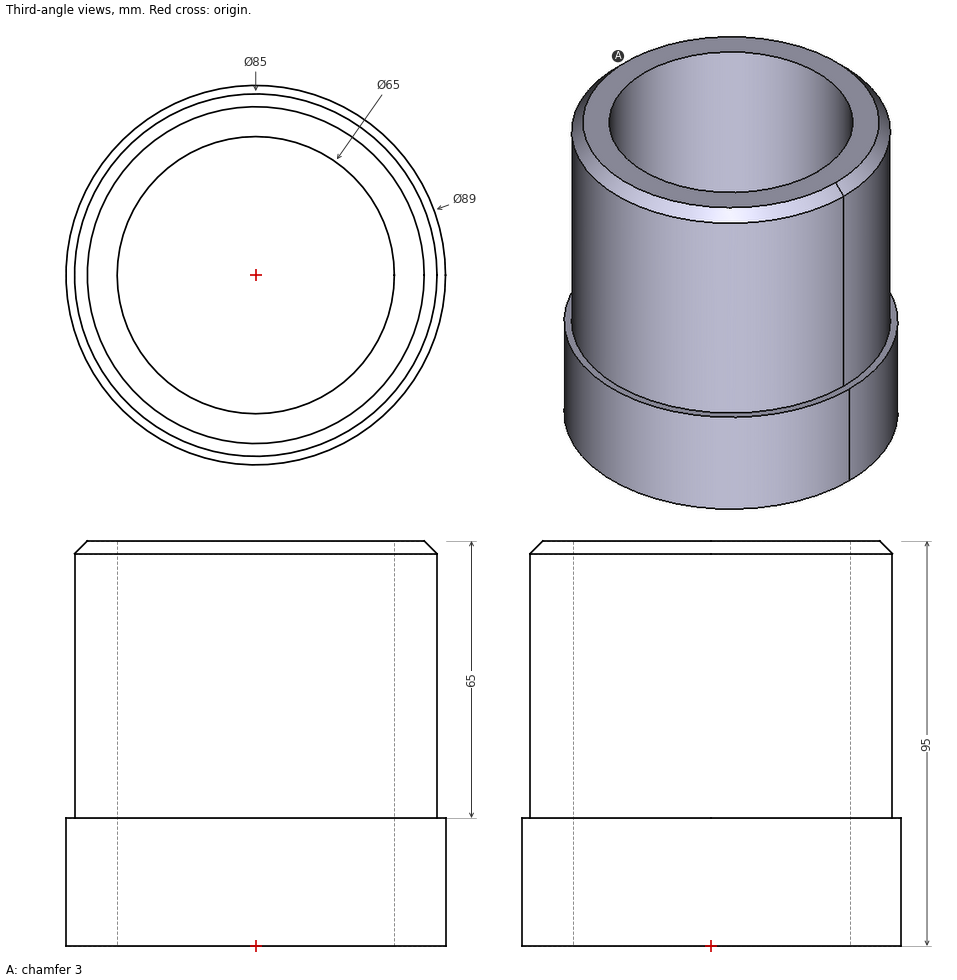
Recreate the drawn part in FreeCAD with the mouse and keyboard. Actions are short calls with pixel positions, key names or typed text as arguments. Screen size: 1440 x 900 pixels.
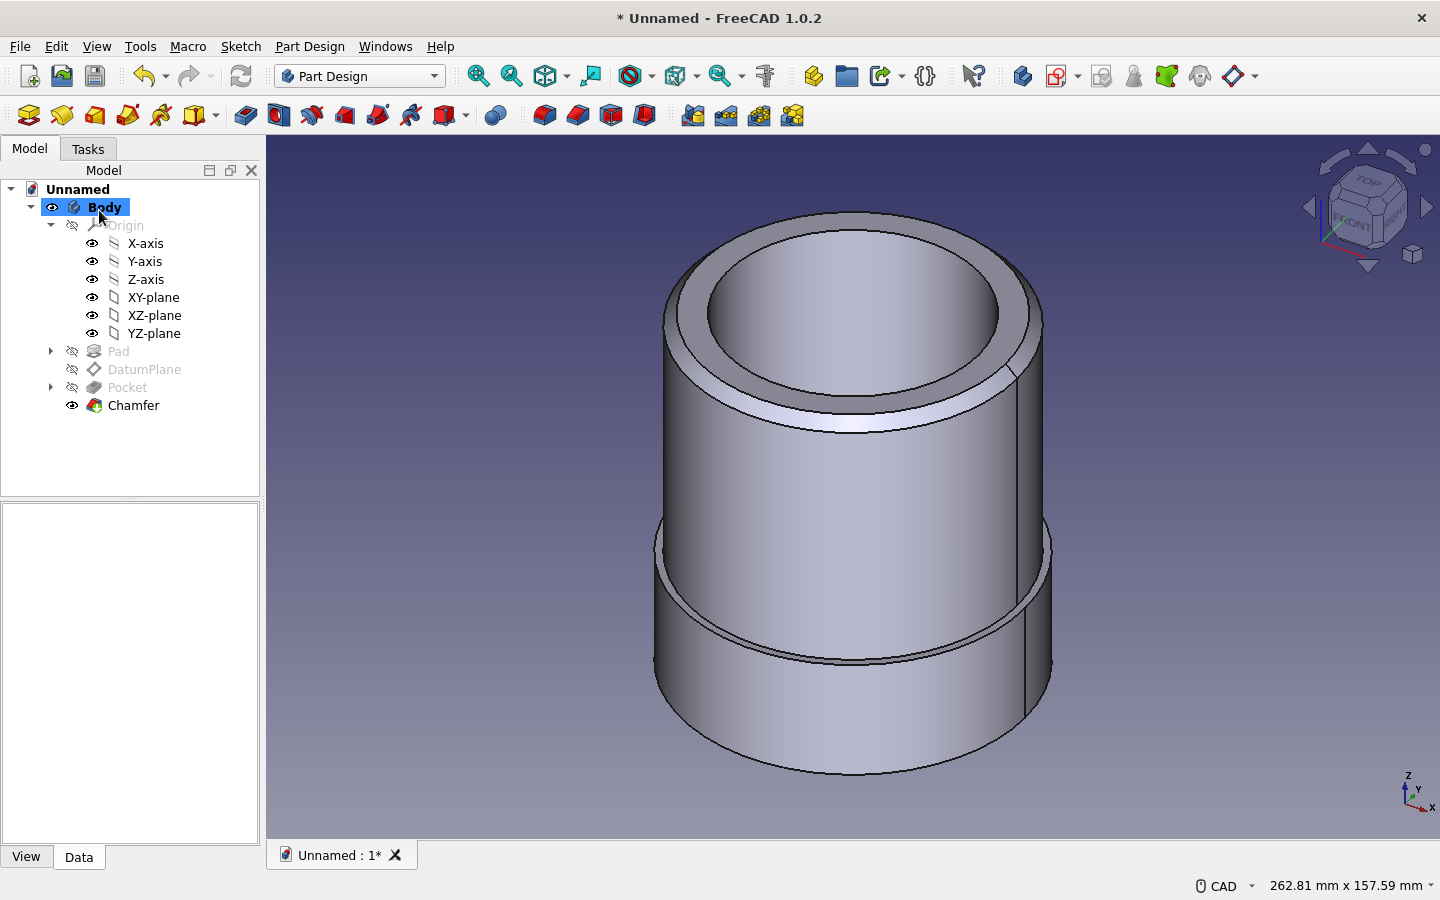
key(0)